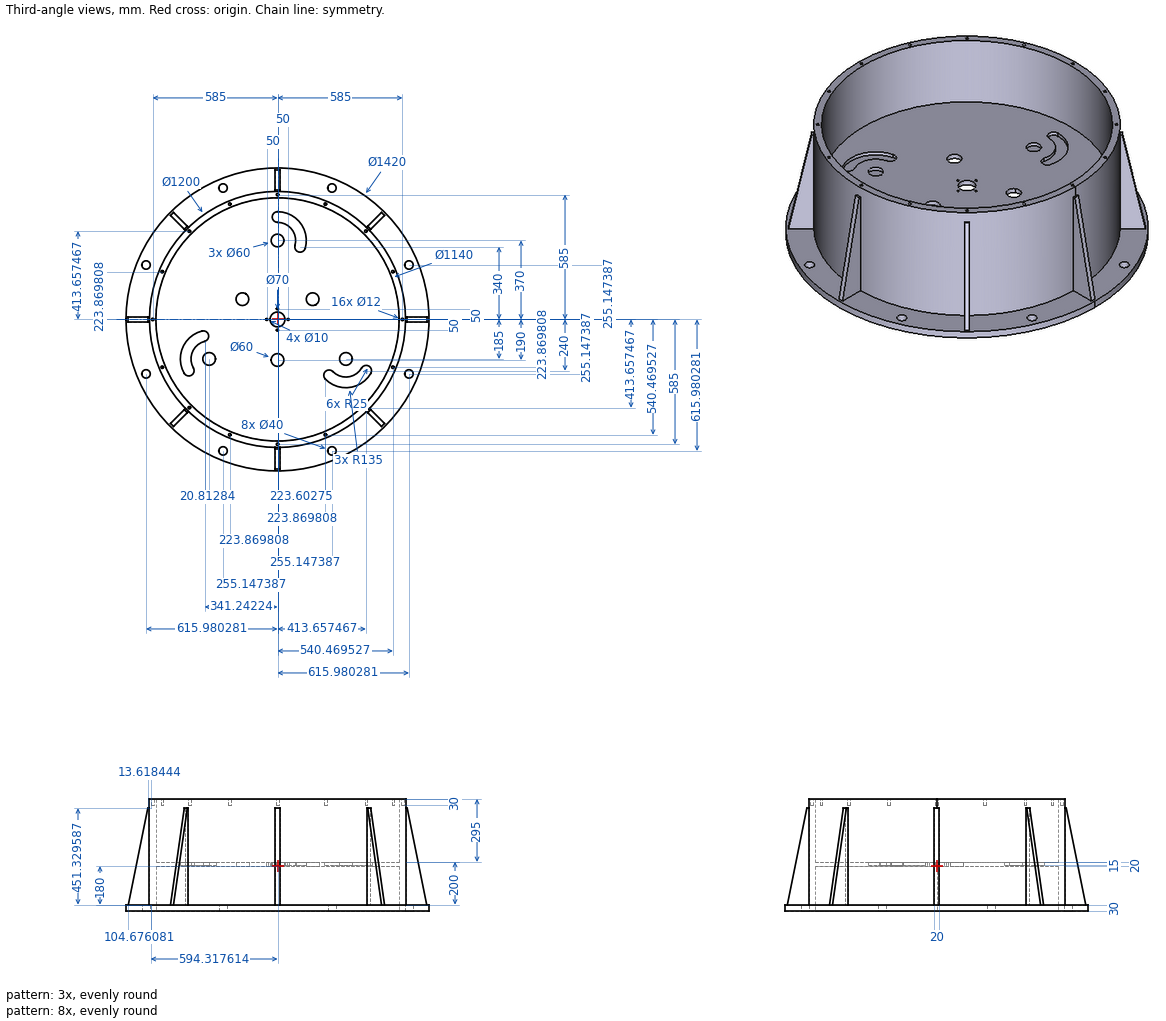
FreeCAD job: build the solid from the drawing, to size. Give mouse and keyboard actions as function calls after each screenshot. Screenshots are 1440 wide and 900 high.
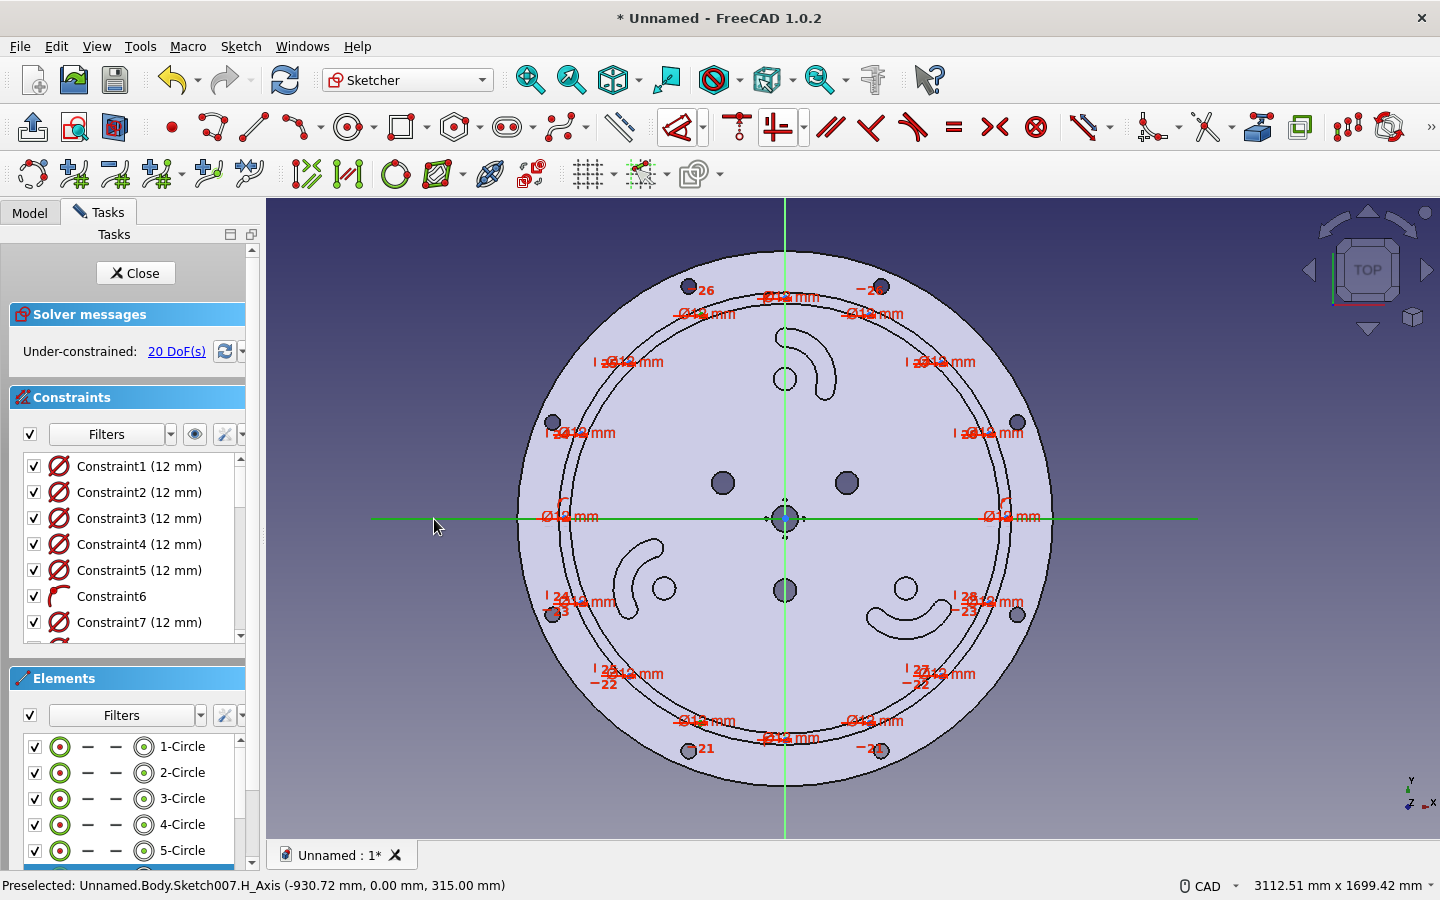
click(995, 128)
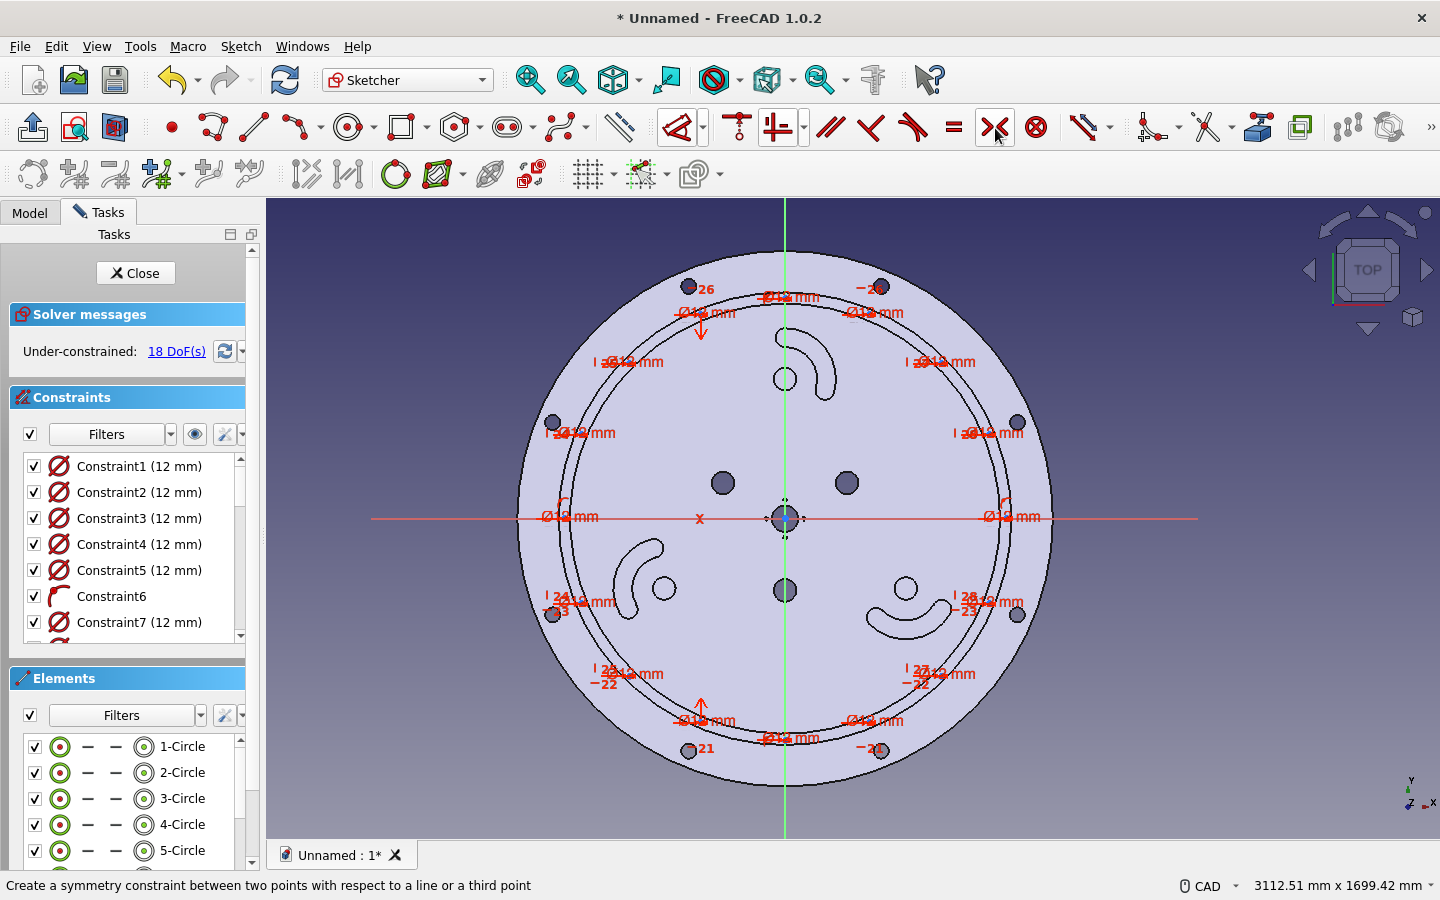
click(629, 364)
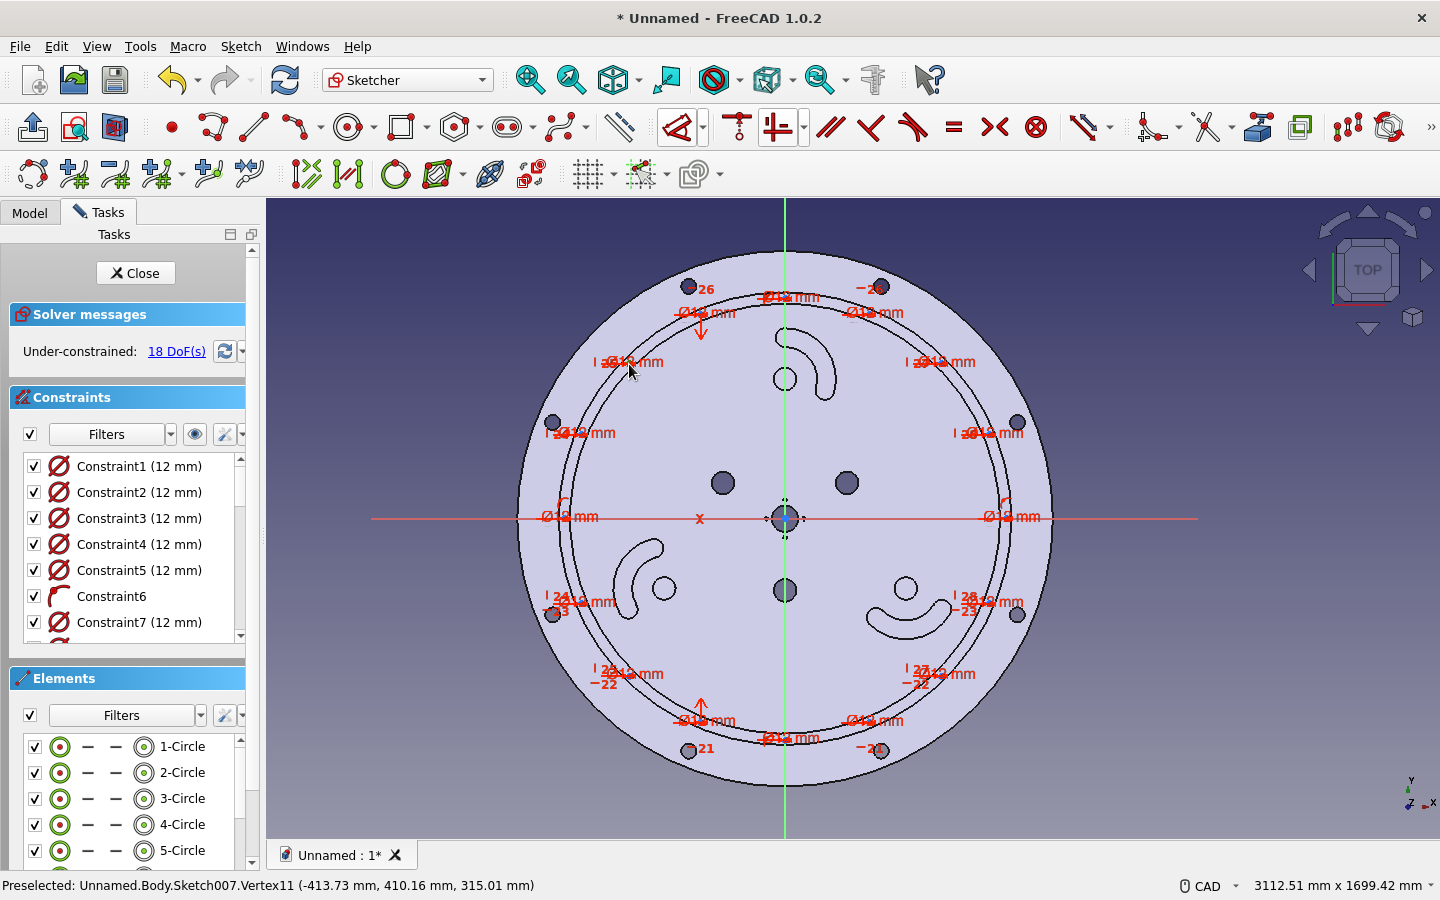
click(941, 364)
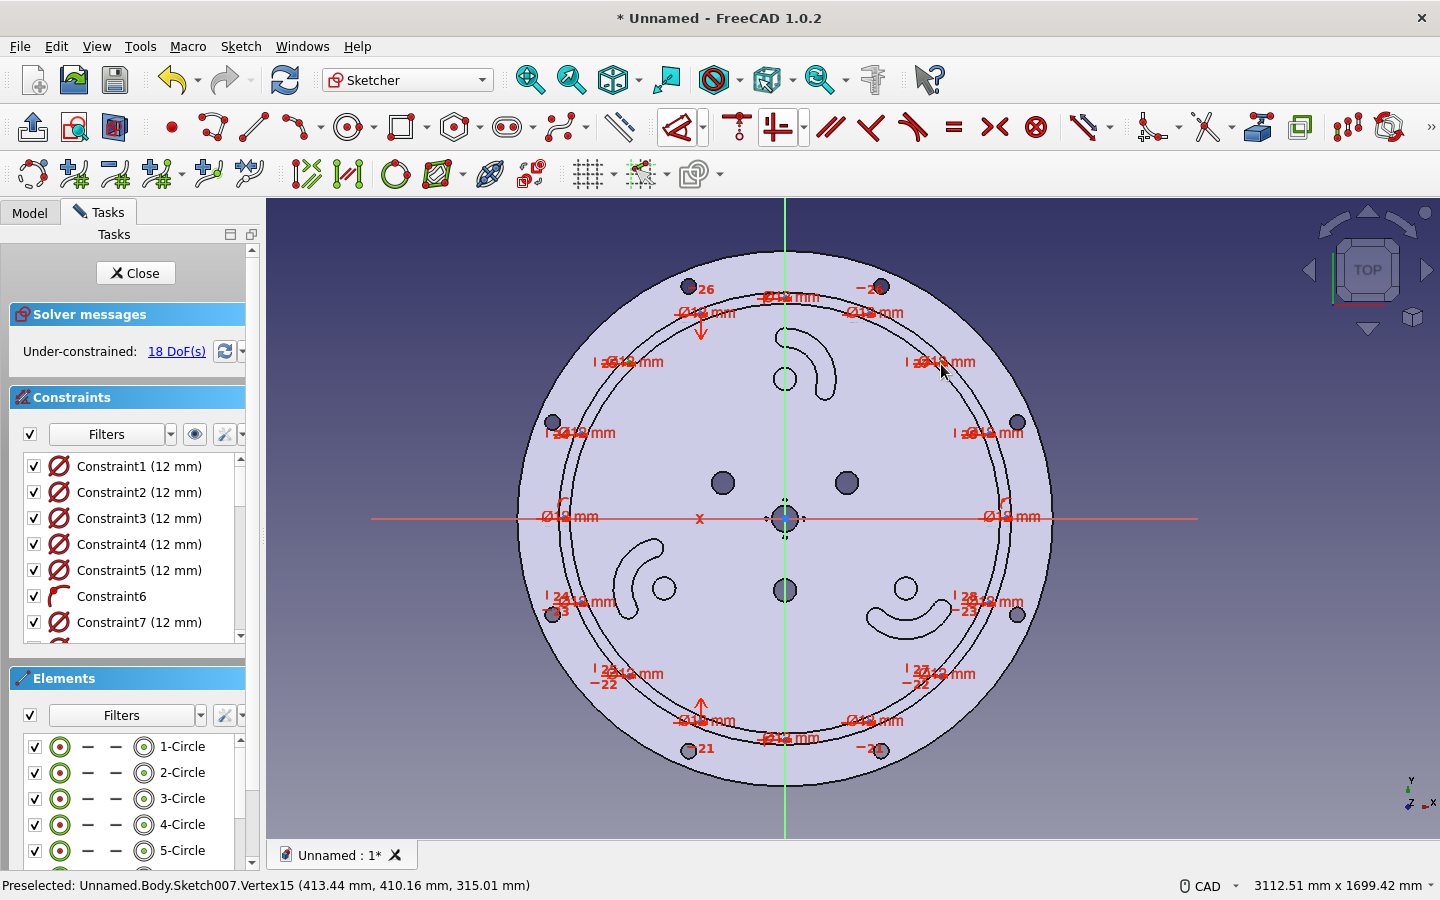
click(785, 686)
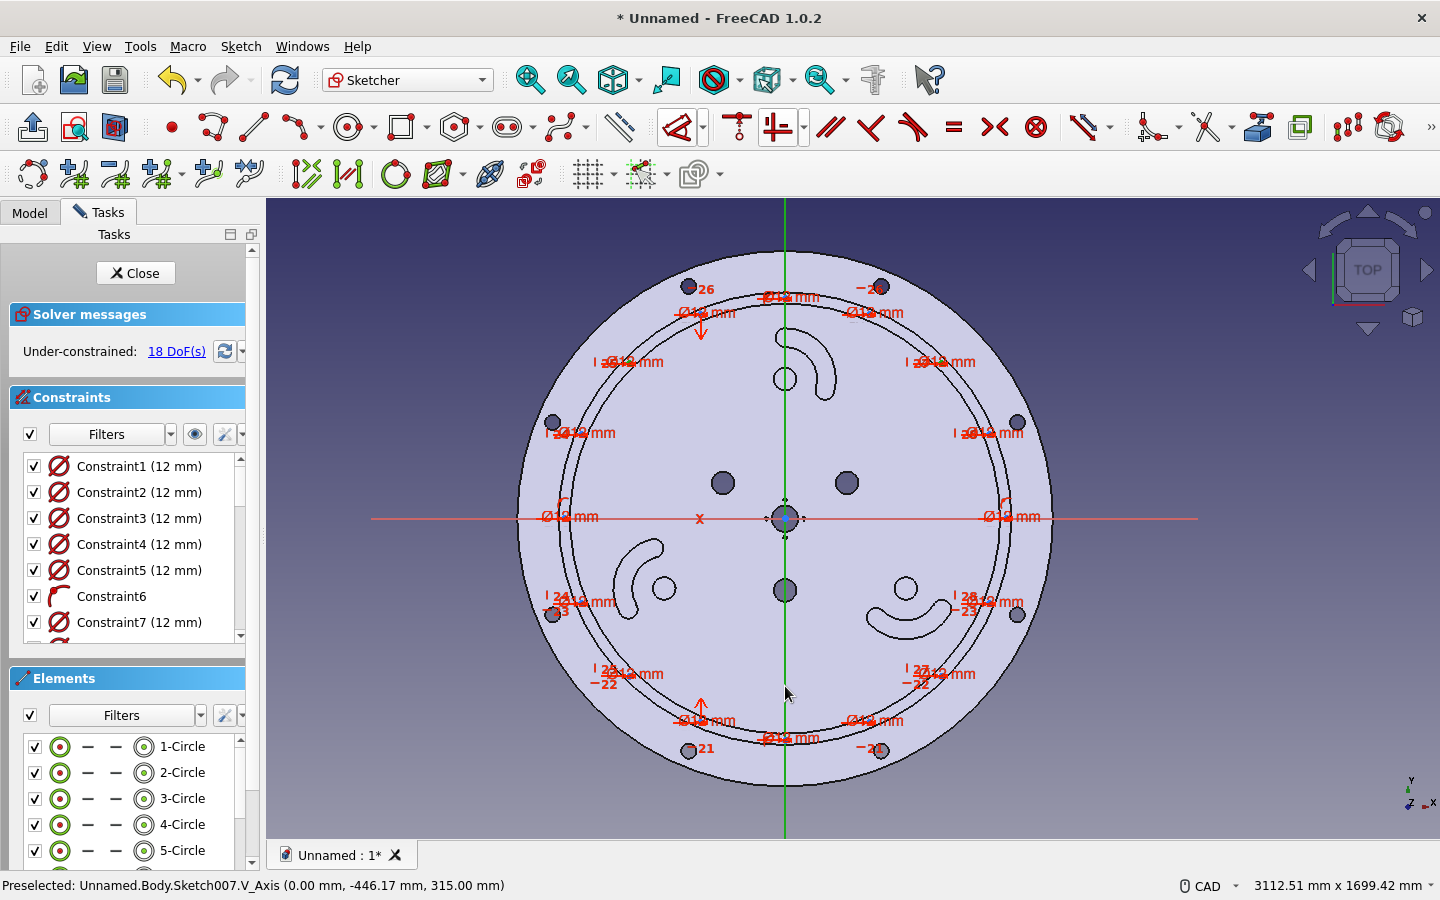
key(s)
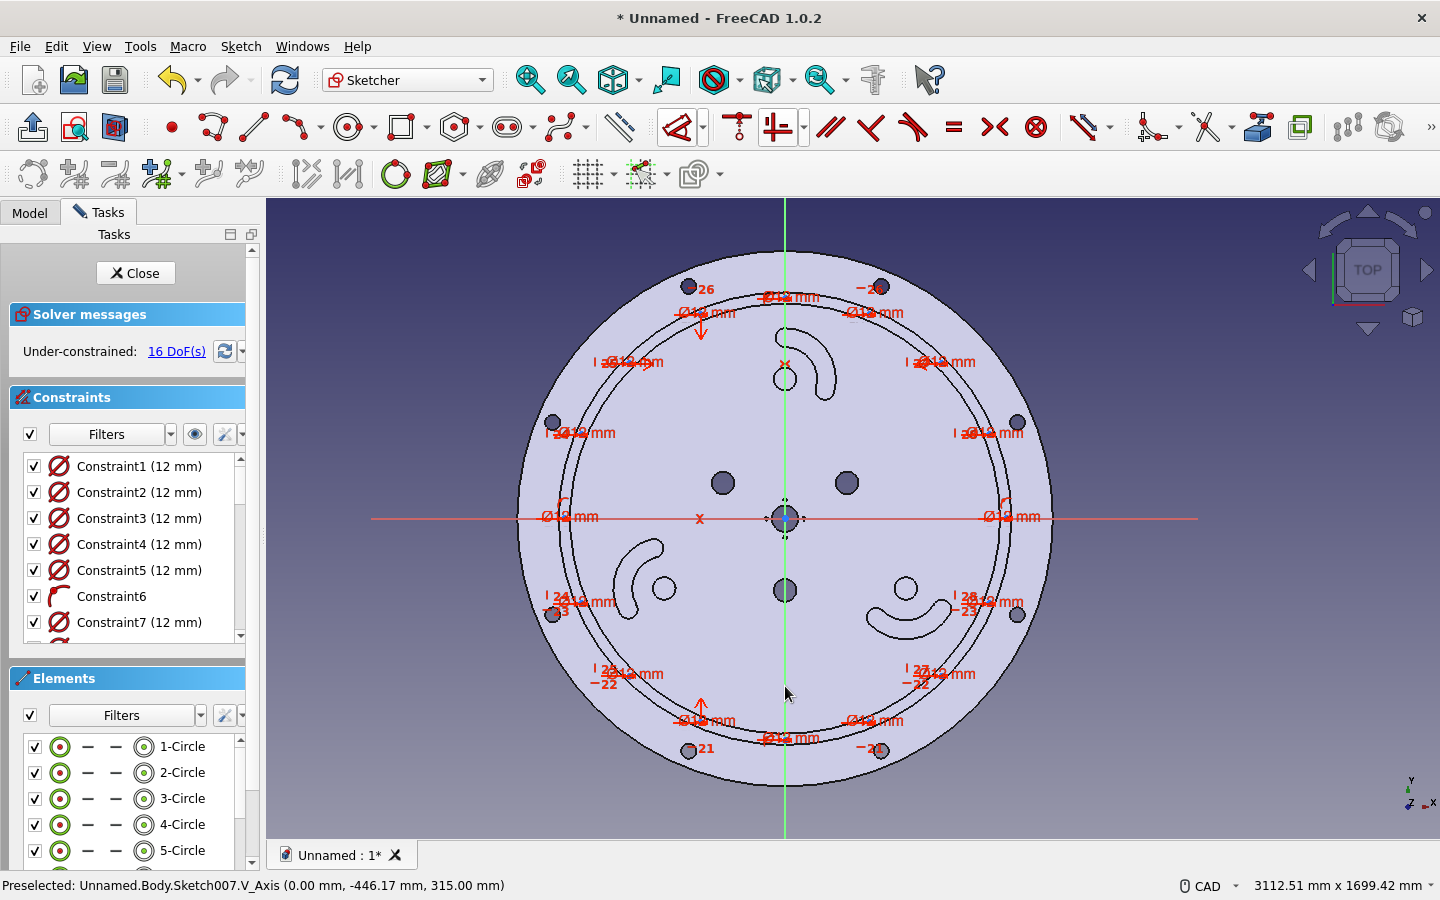
click(581, 435)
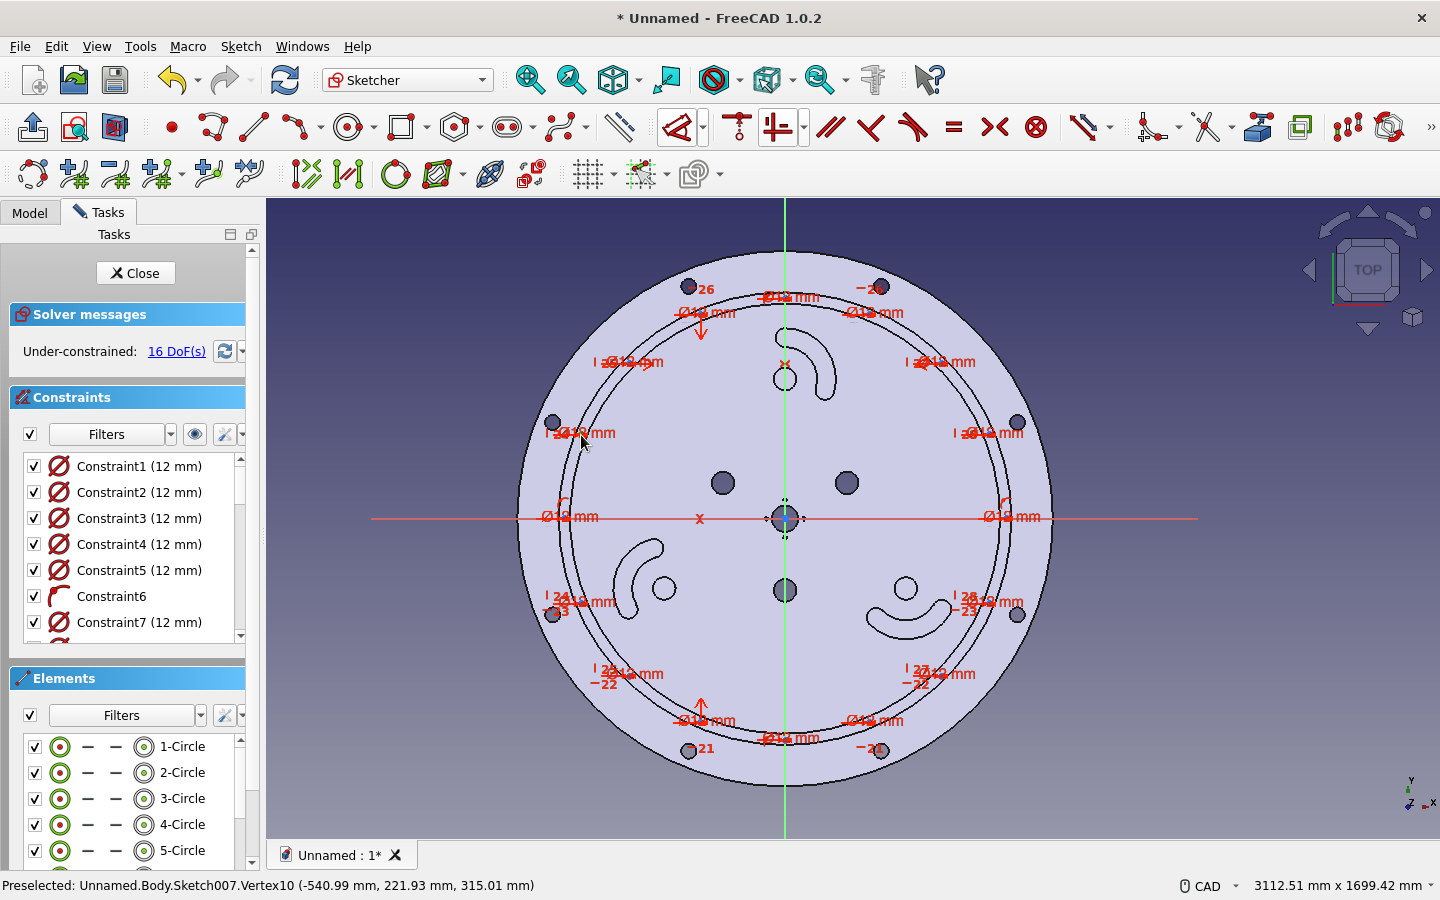
click(989, 435)